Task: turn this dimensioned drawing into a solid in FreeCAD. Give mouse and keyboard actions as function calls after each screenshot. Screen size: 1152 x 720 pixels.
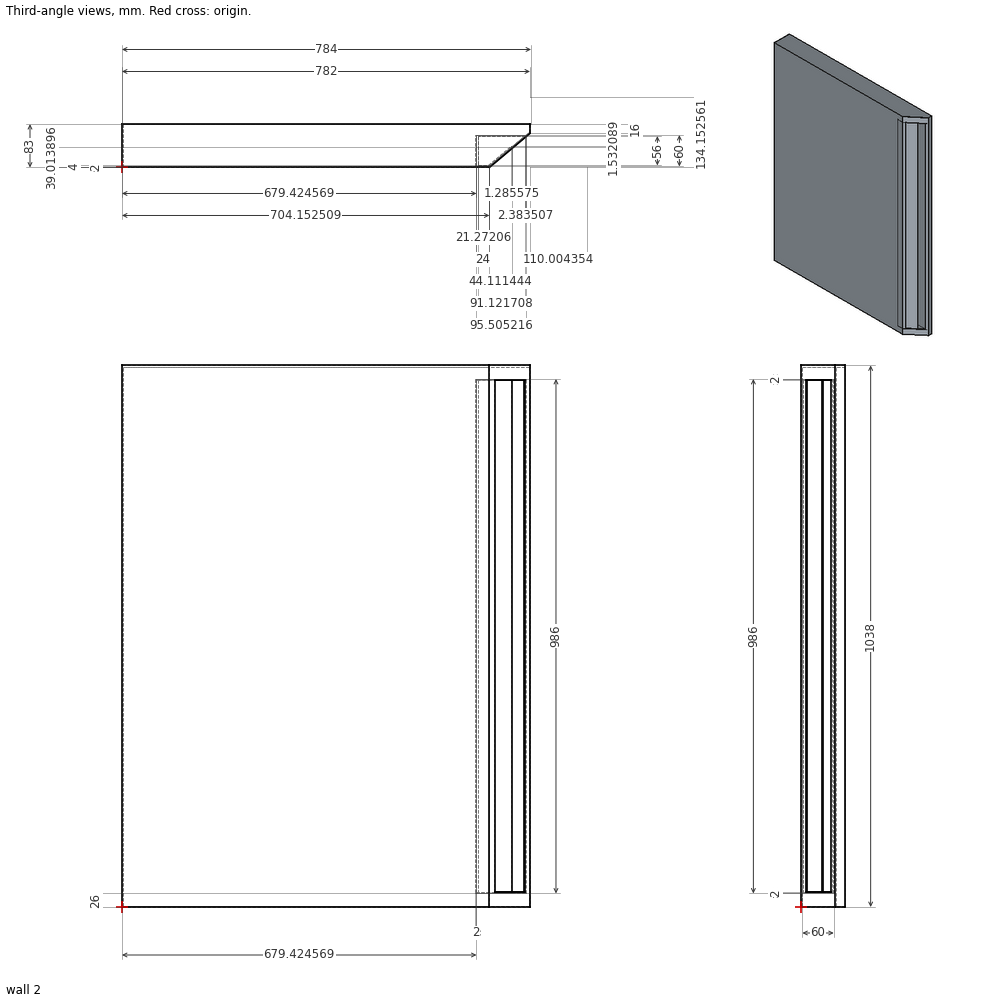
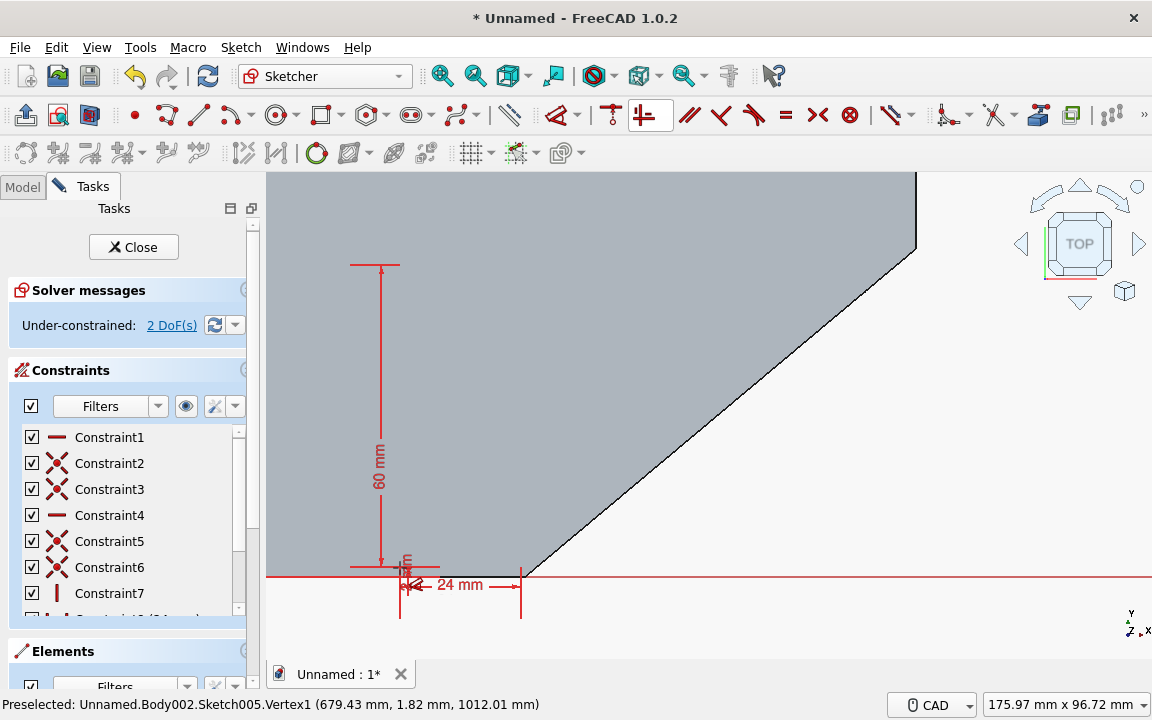
click(737, 265)
click(641, 231)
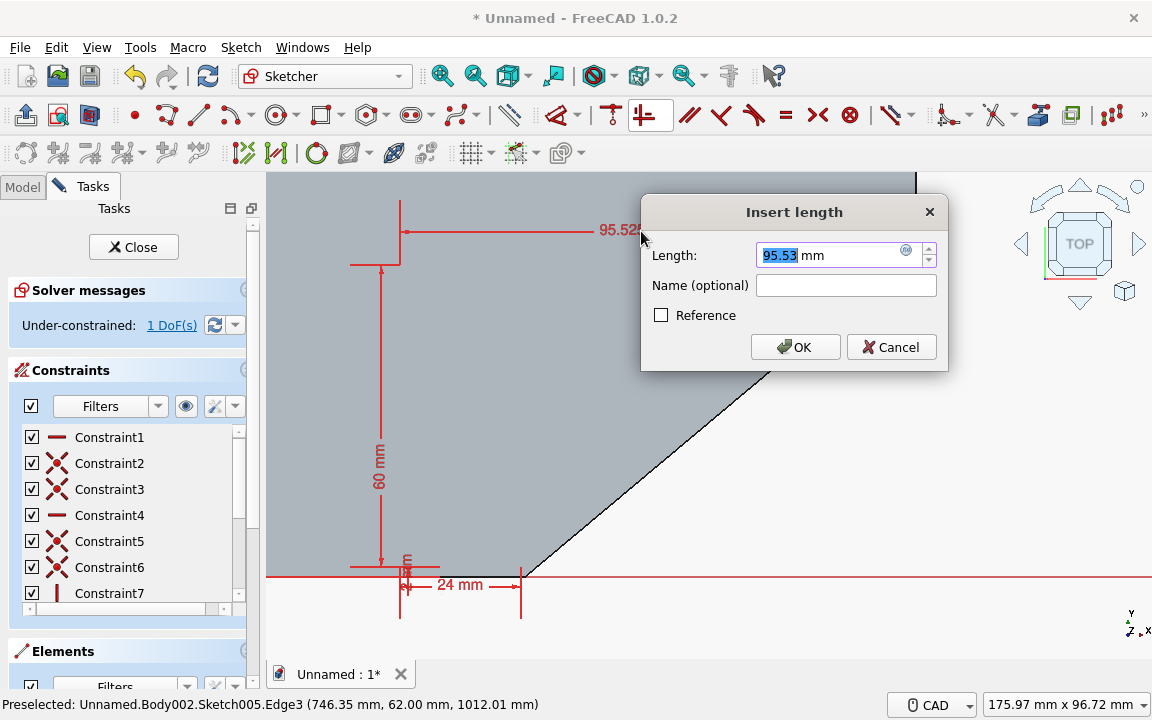
text(95.505216)
key(Return)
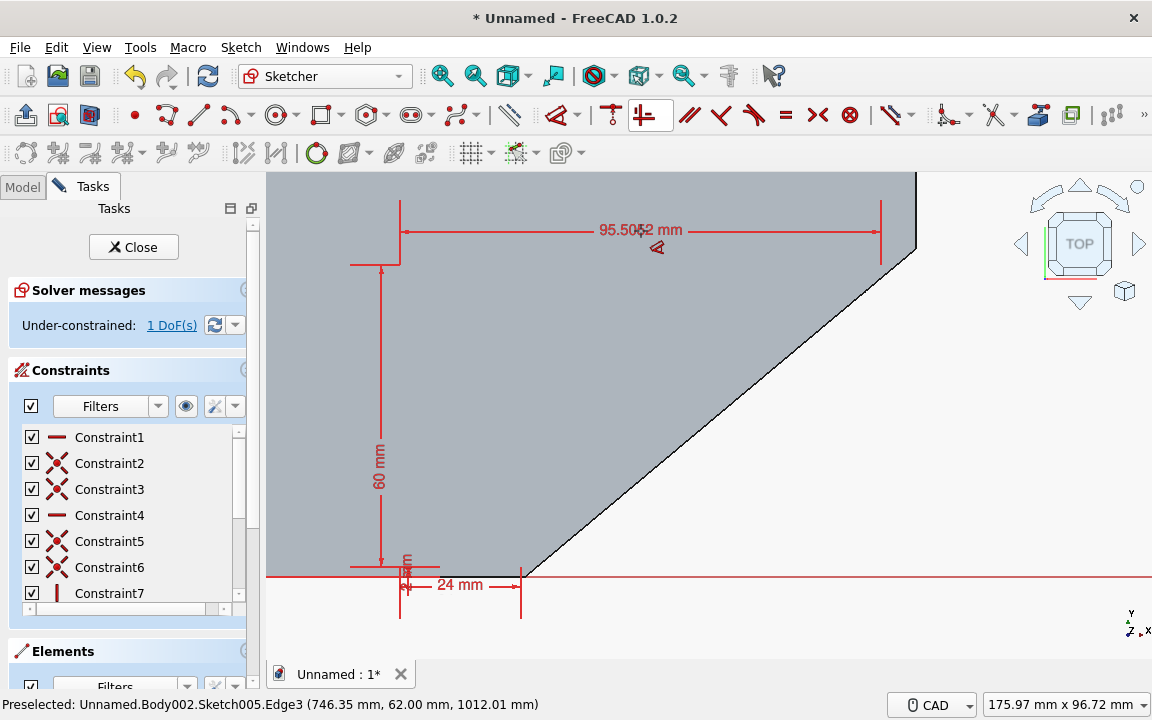
click(400, 567)
click(347, 611)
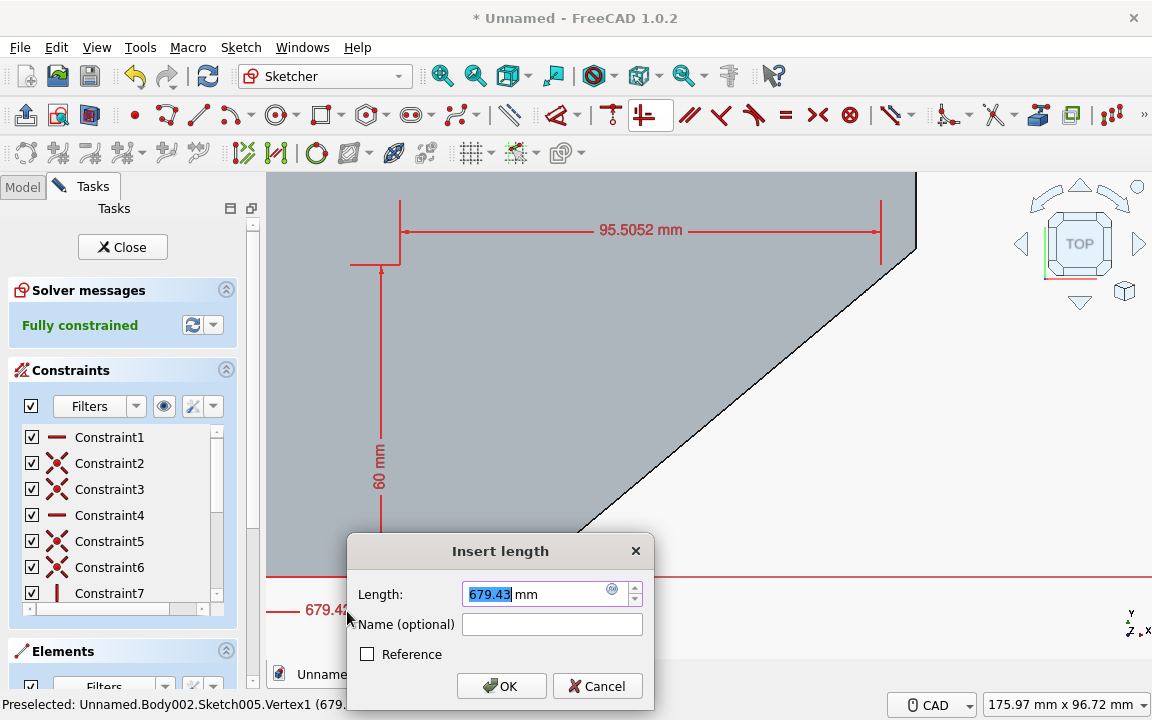
text(679.424569)
key(Return)
key(Escape)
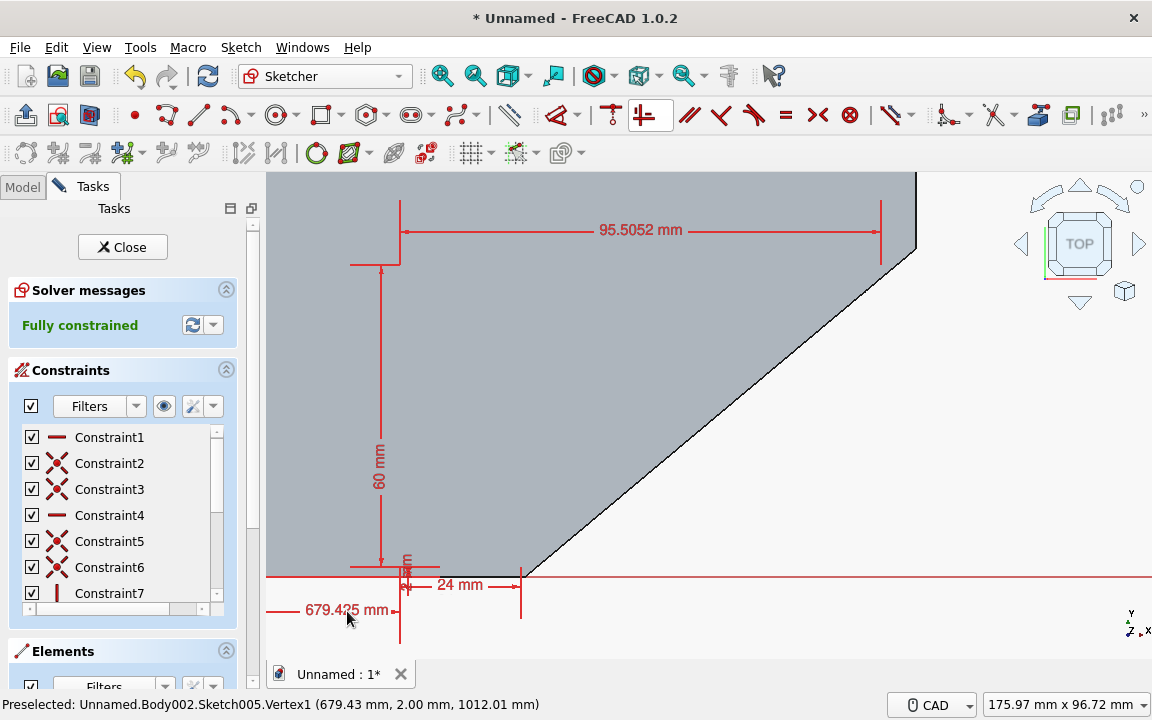
click(123, 247)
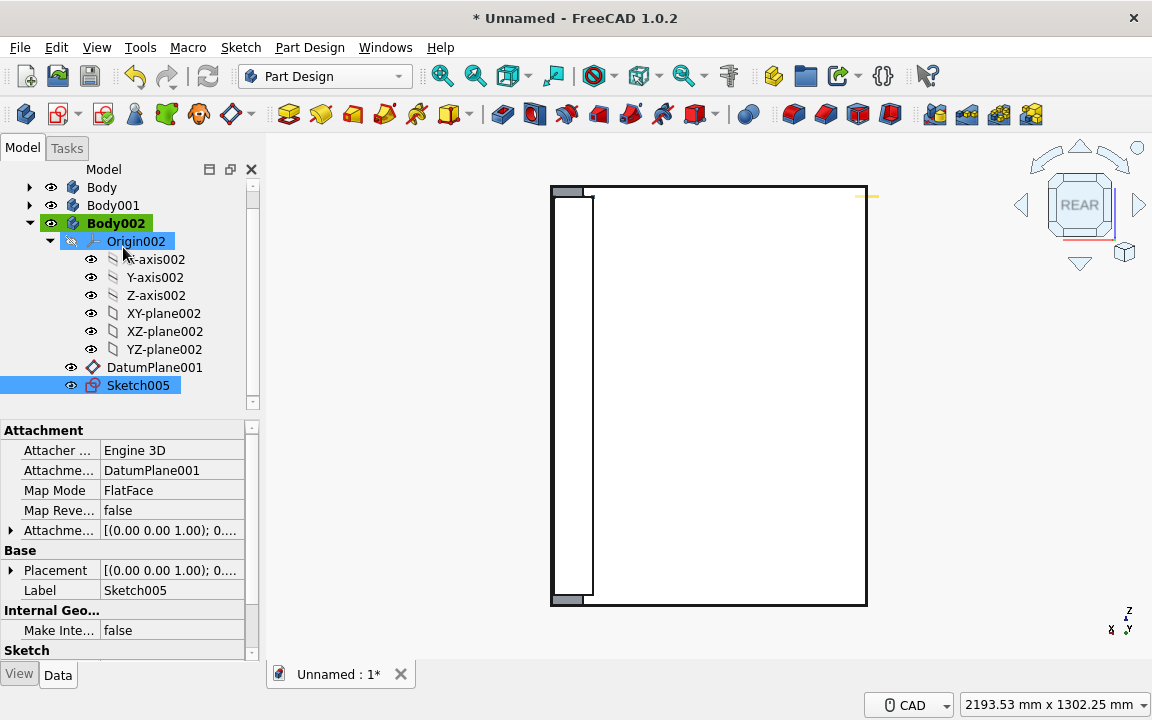
click(290, 114)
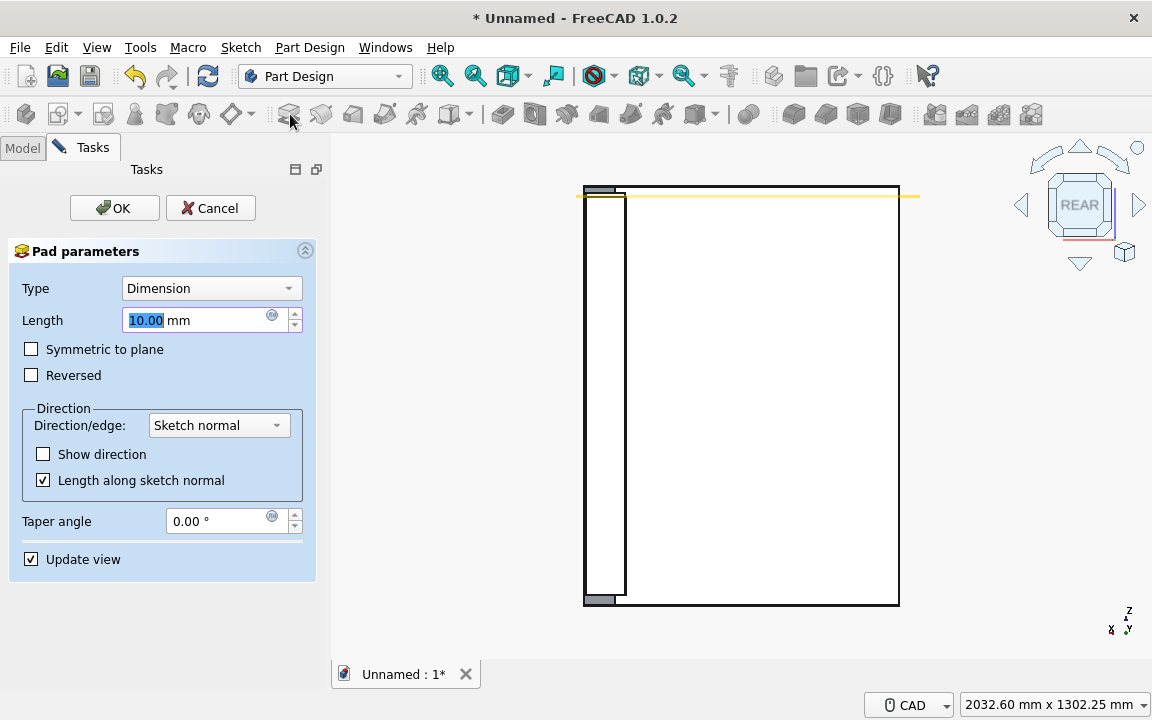
text(2)
key(Tab)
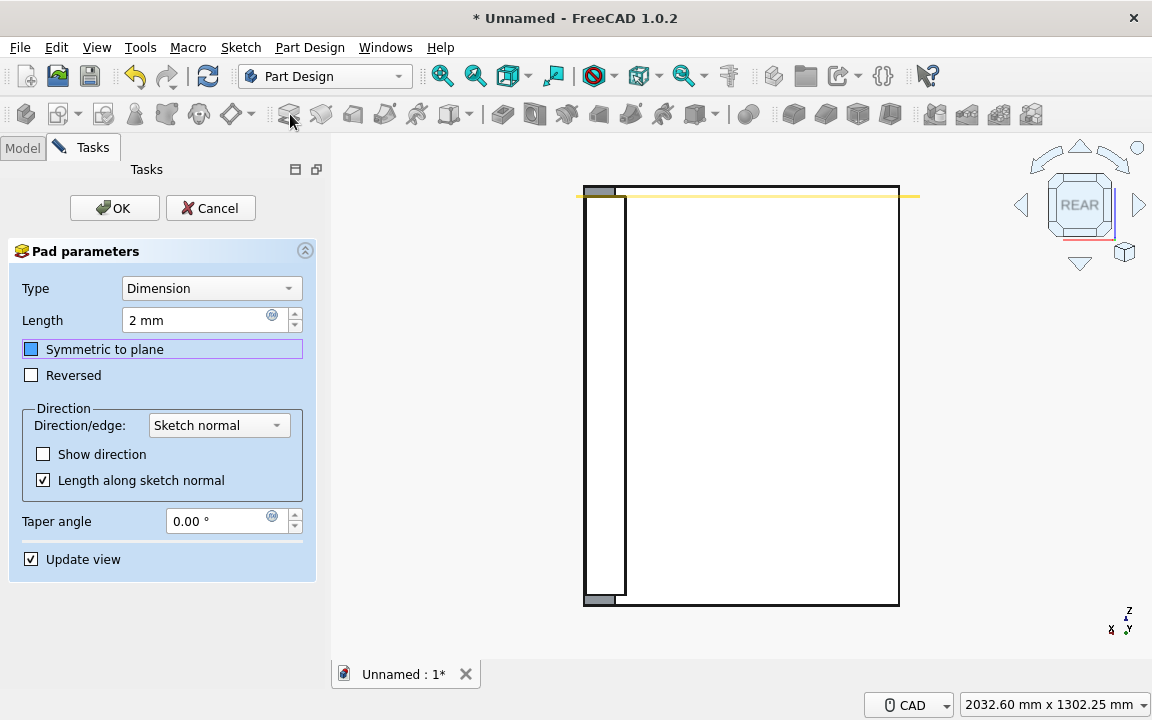
click(30, 375)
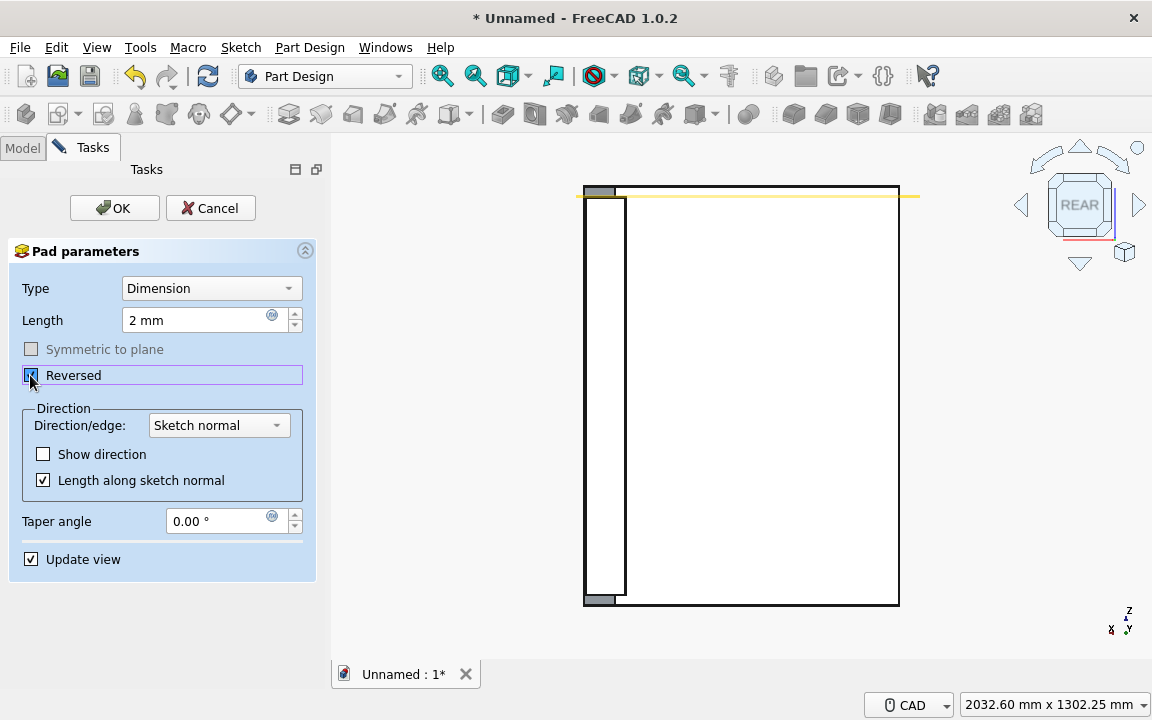
click(115, 208)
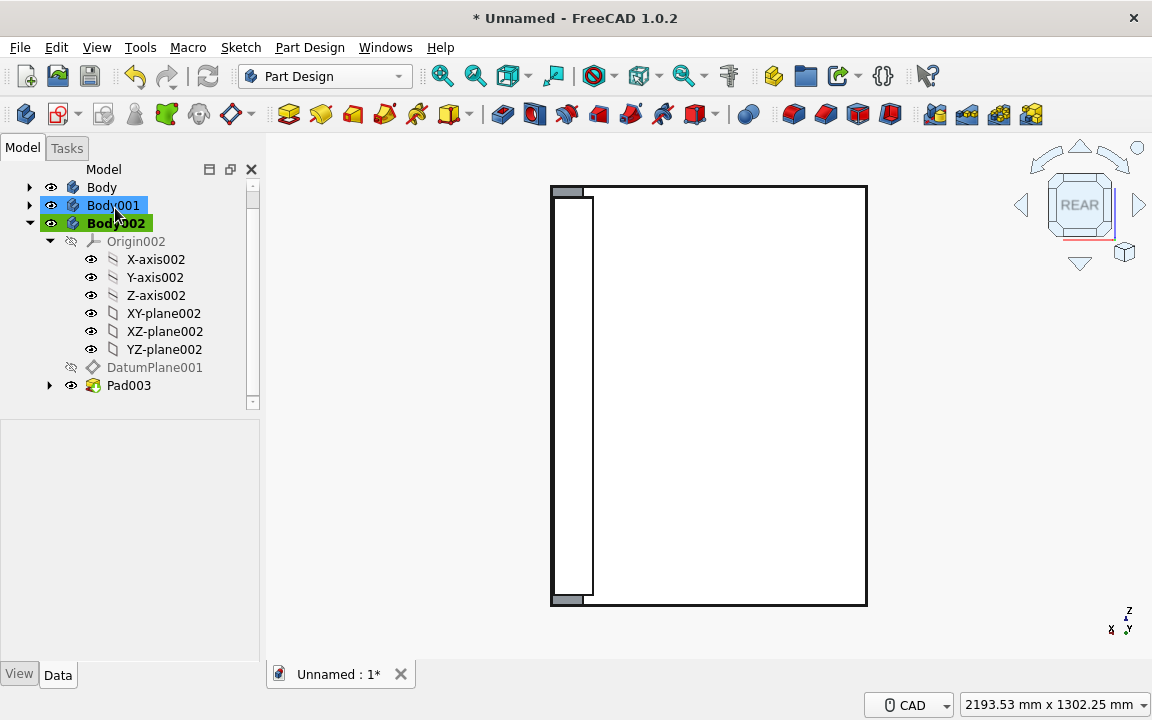
key(v)
key(f)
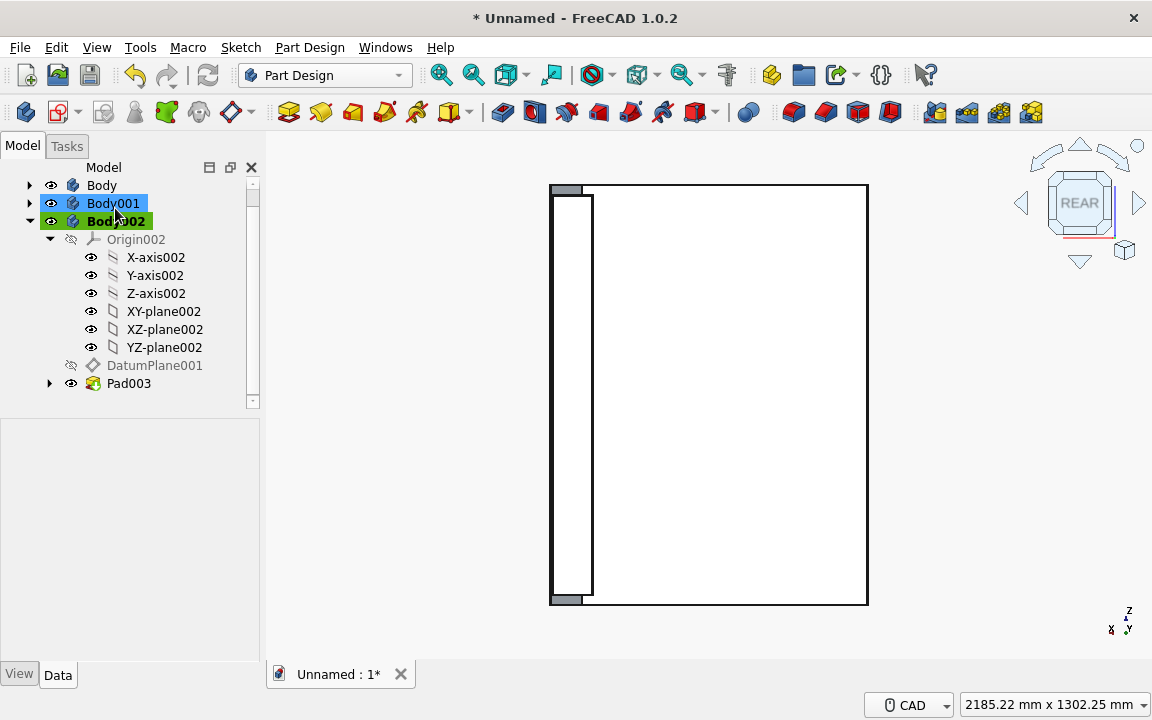
click(26, 112)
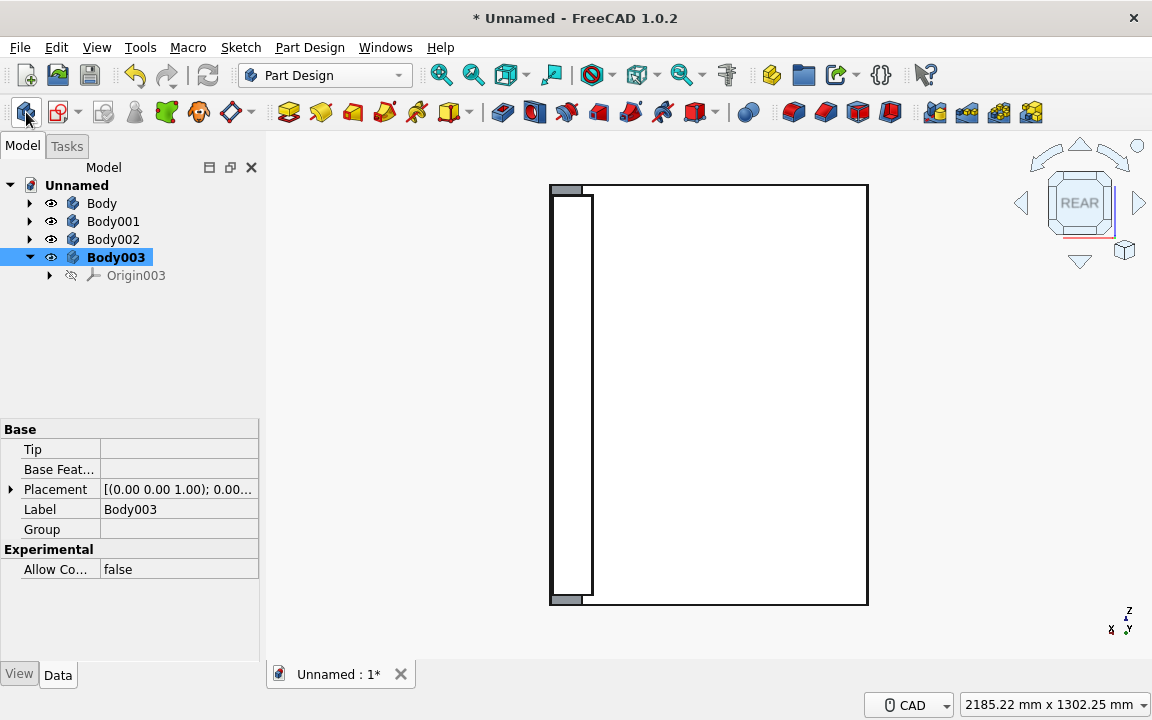
click(50, 275)